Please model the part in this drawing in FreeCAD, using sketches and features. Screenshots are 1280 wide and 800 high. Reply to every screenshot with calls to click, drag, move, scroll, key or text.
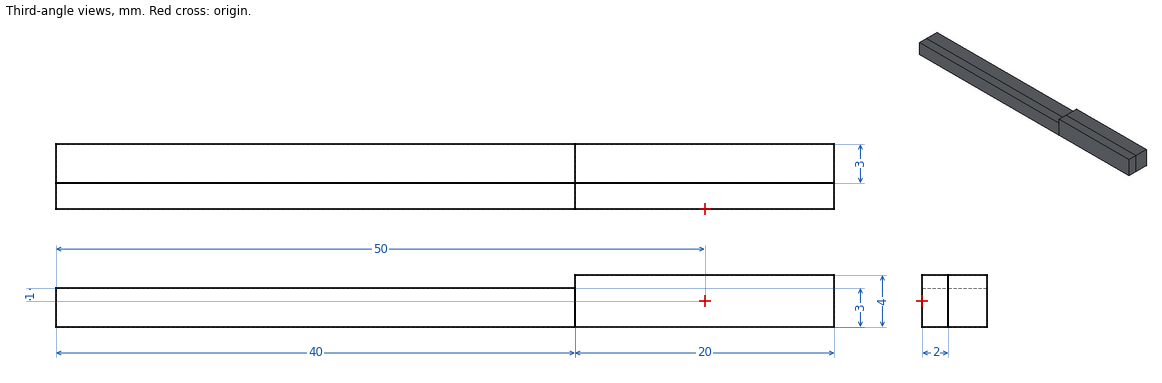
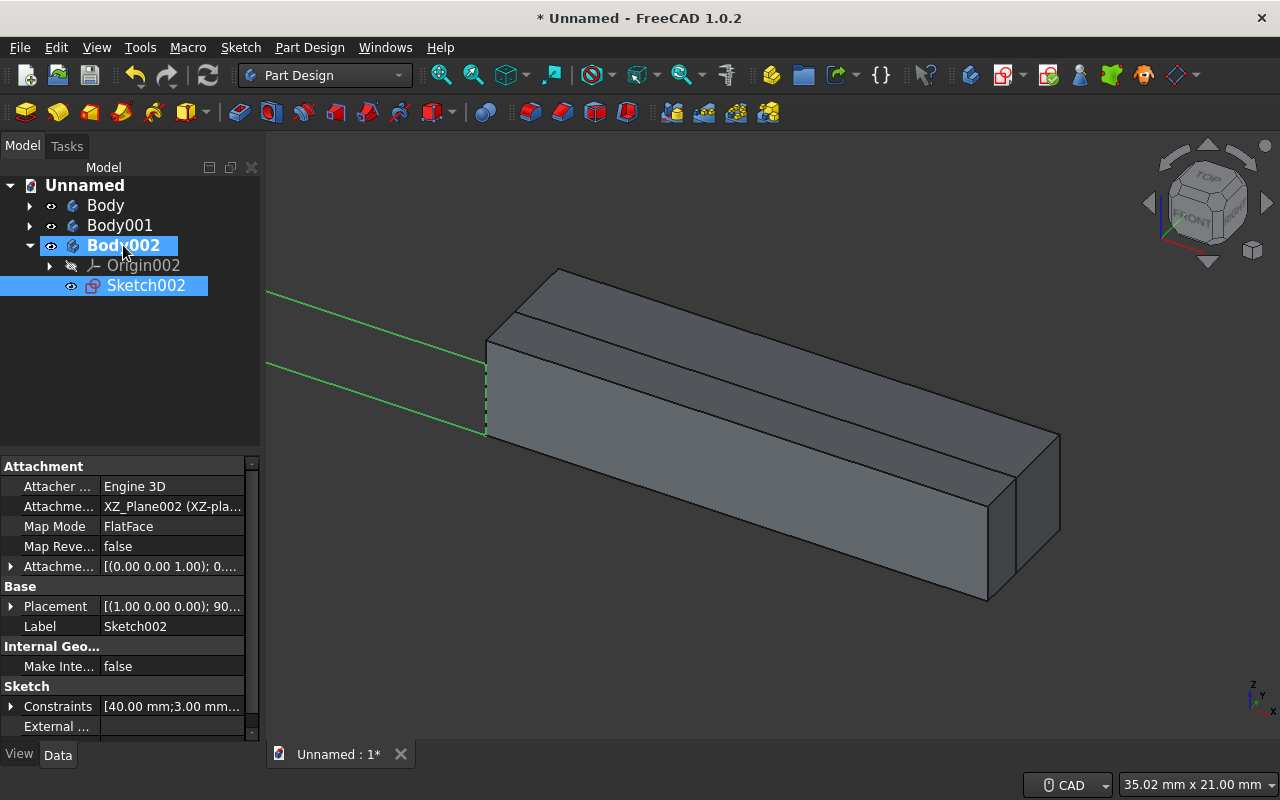
click(26, 112)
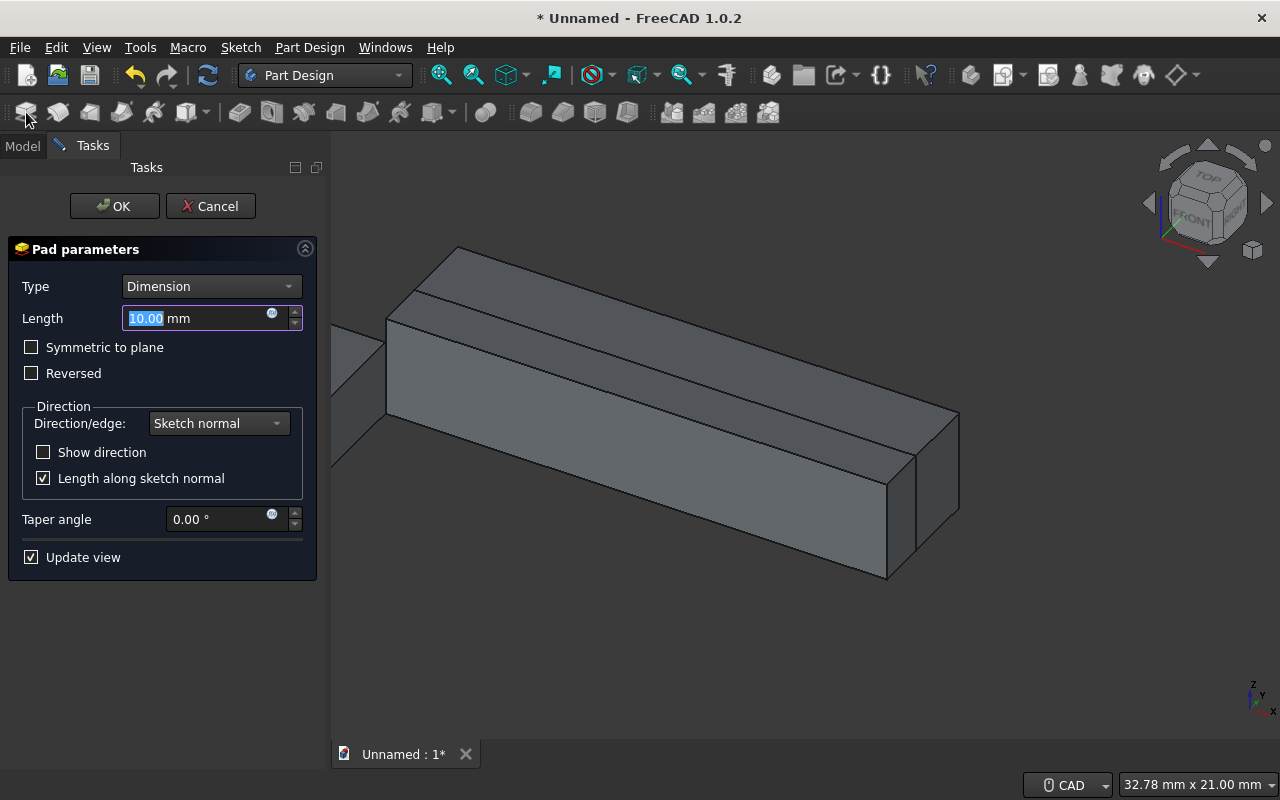
text(2)
key(Tab)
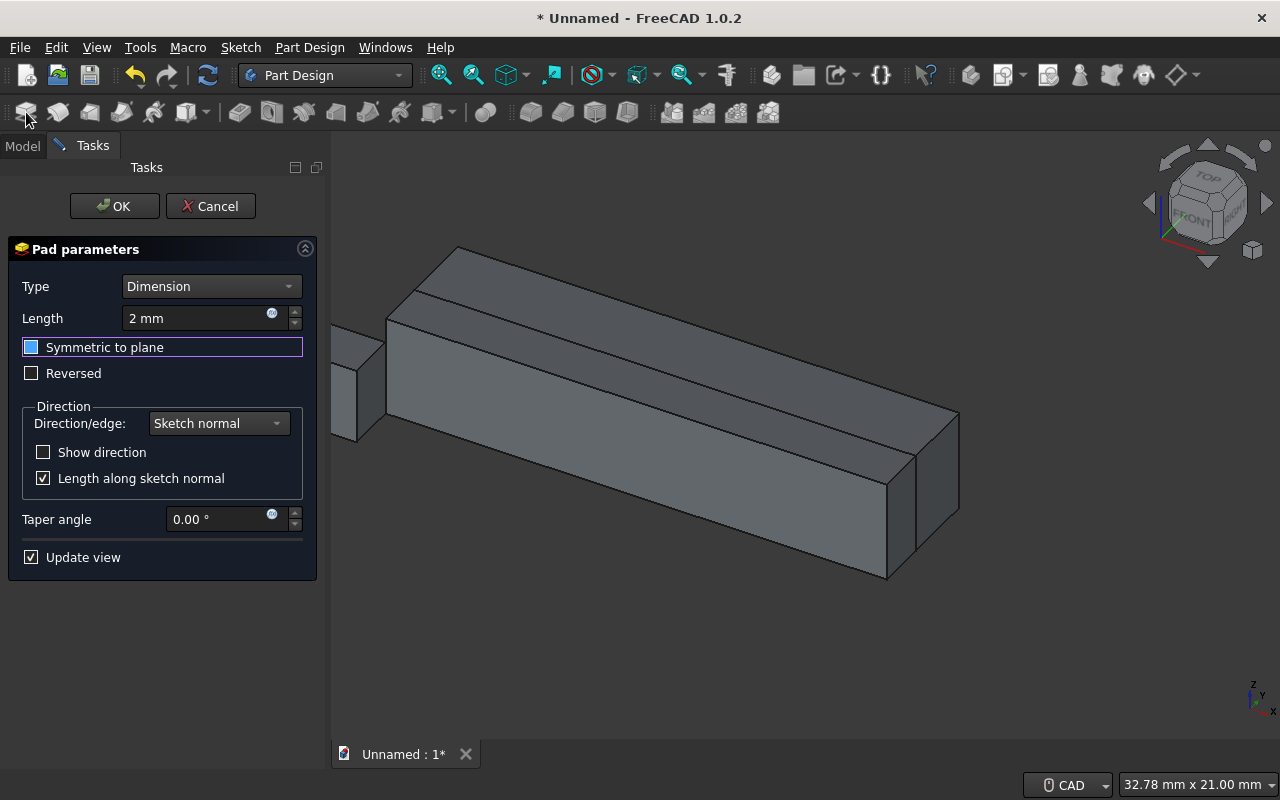
click(30, 373)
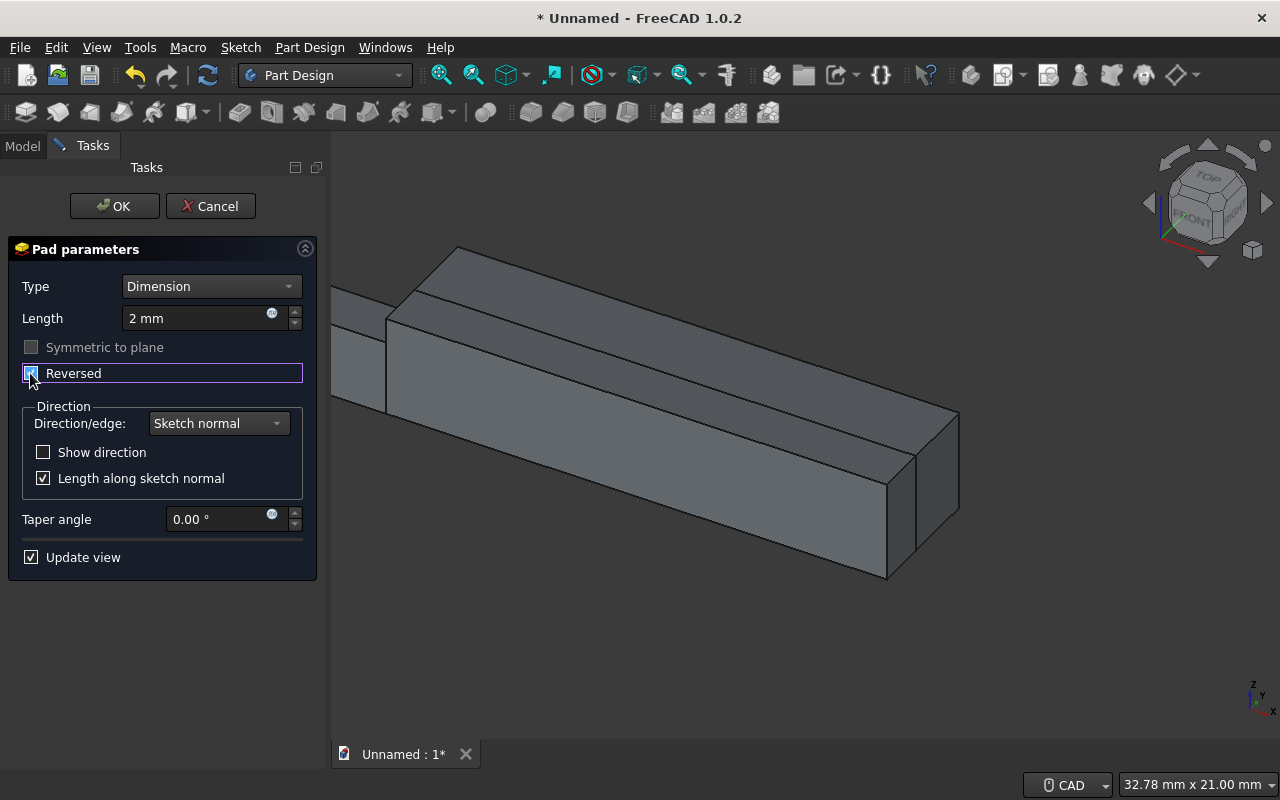
click(115, 206)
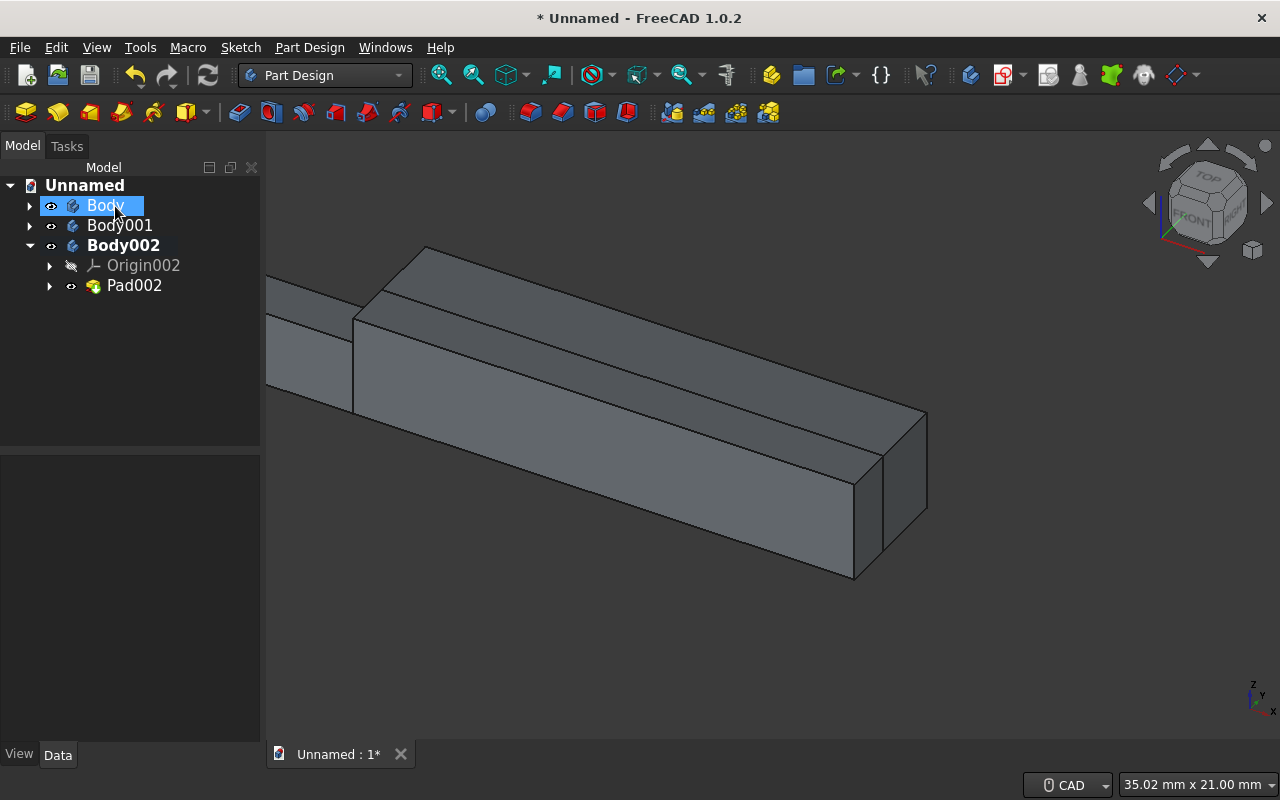
click(442, 76)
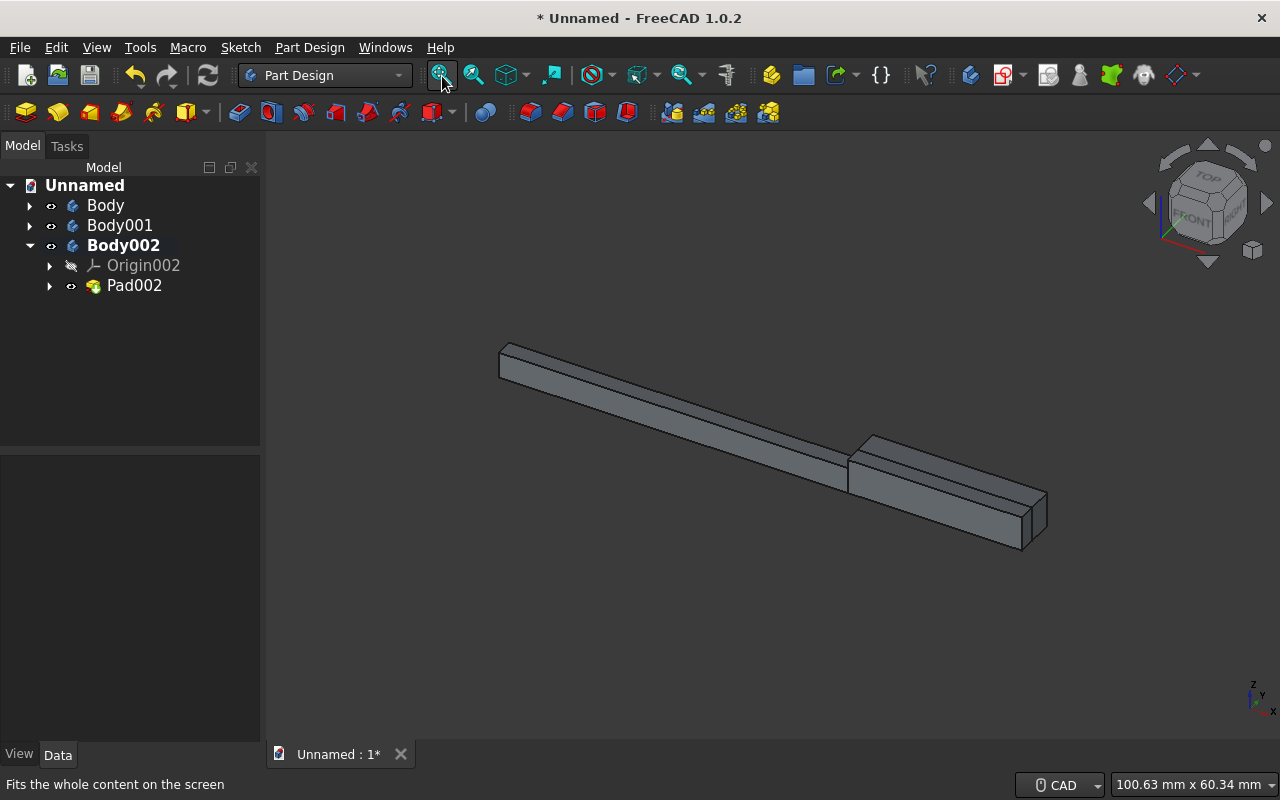
click(972, 76)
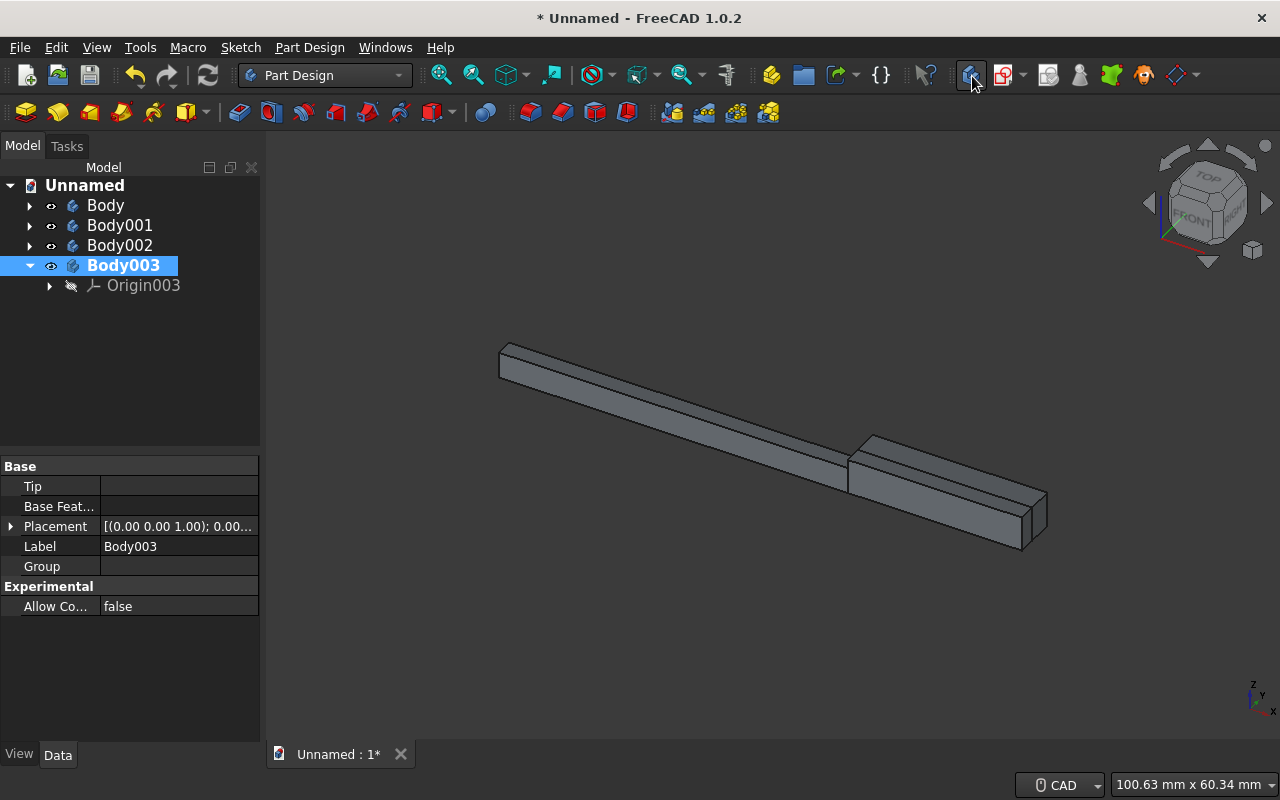
click(50, 286)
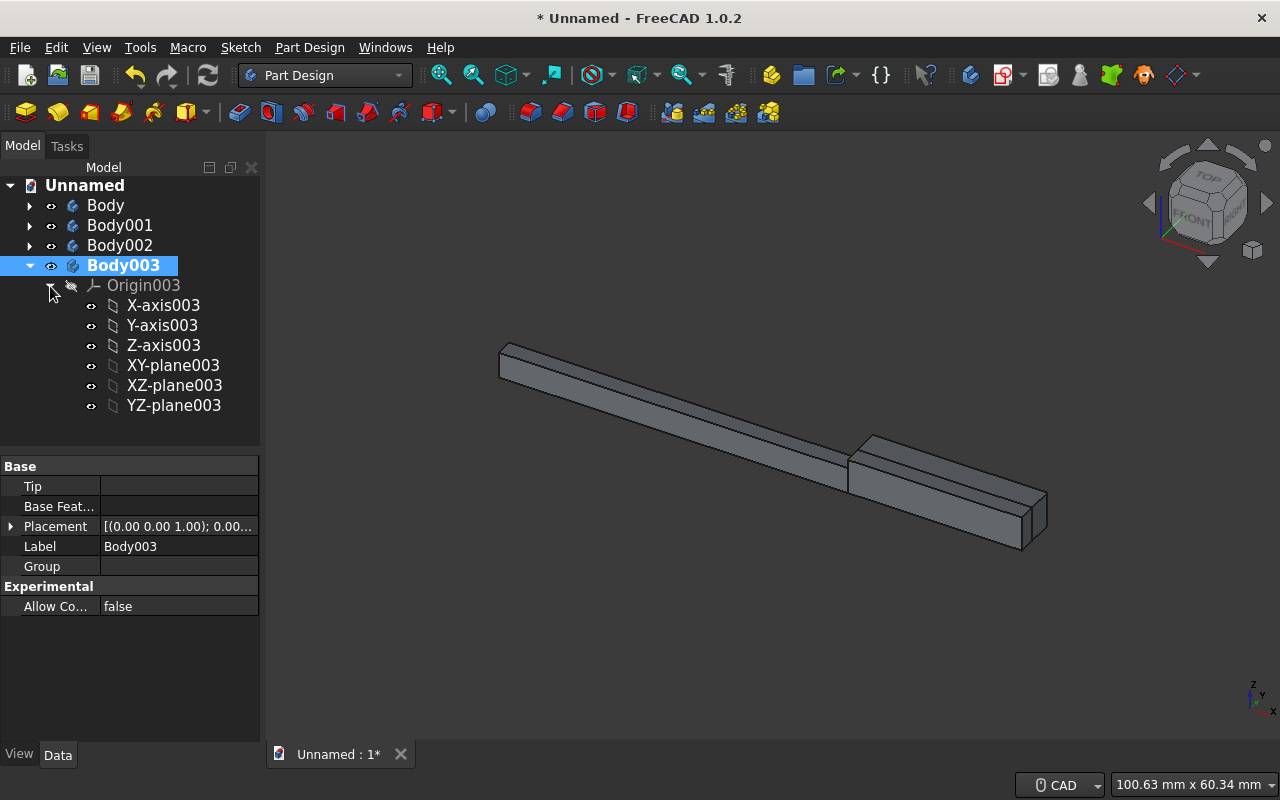
click(136, 386)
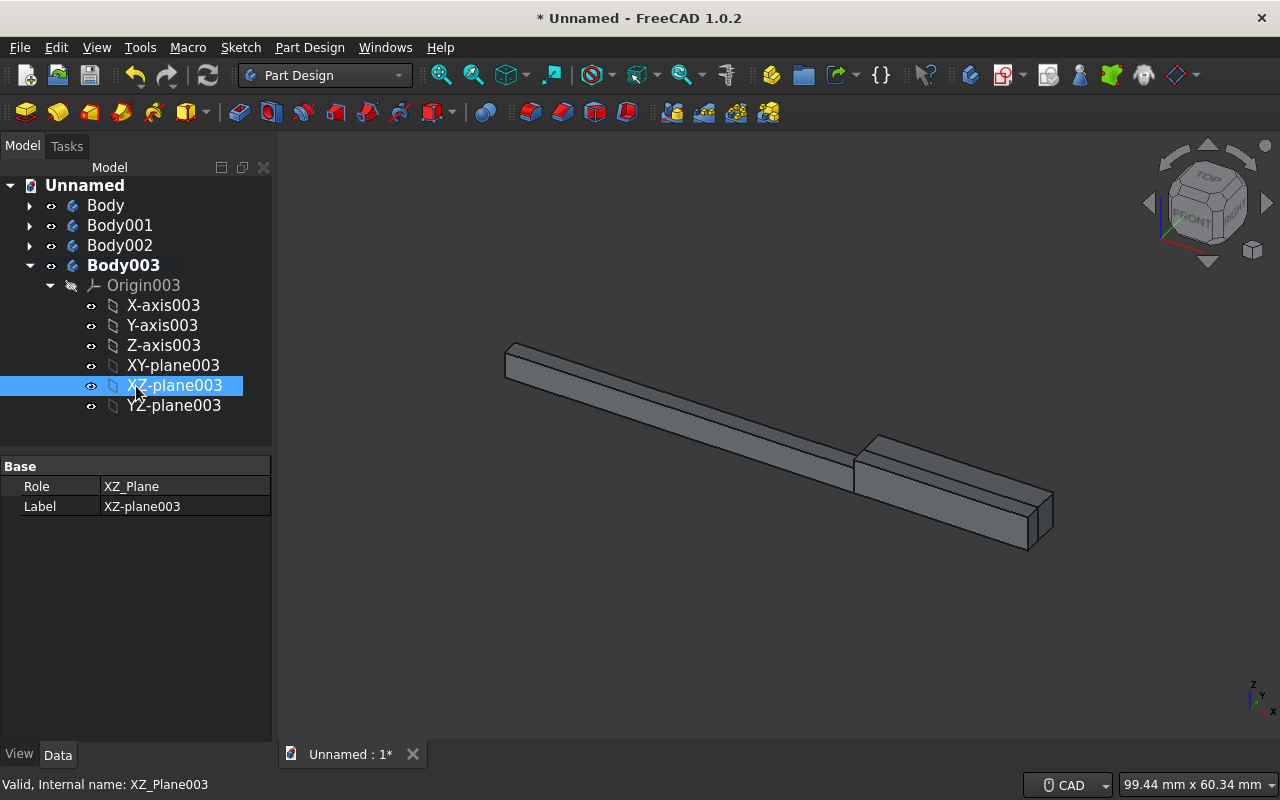
click(1176, 76)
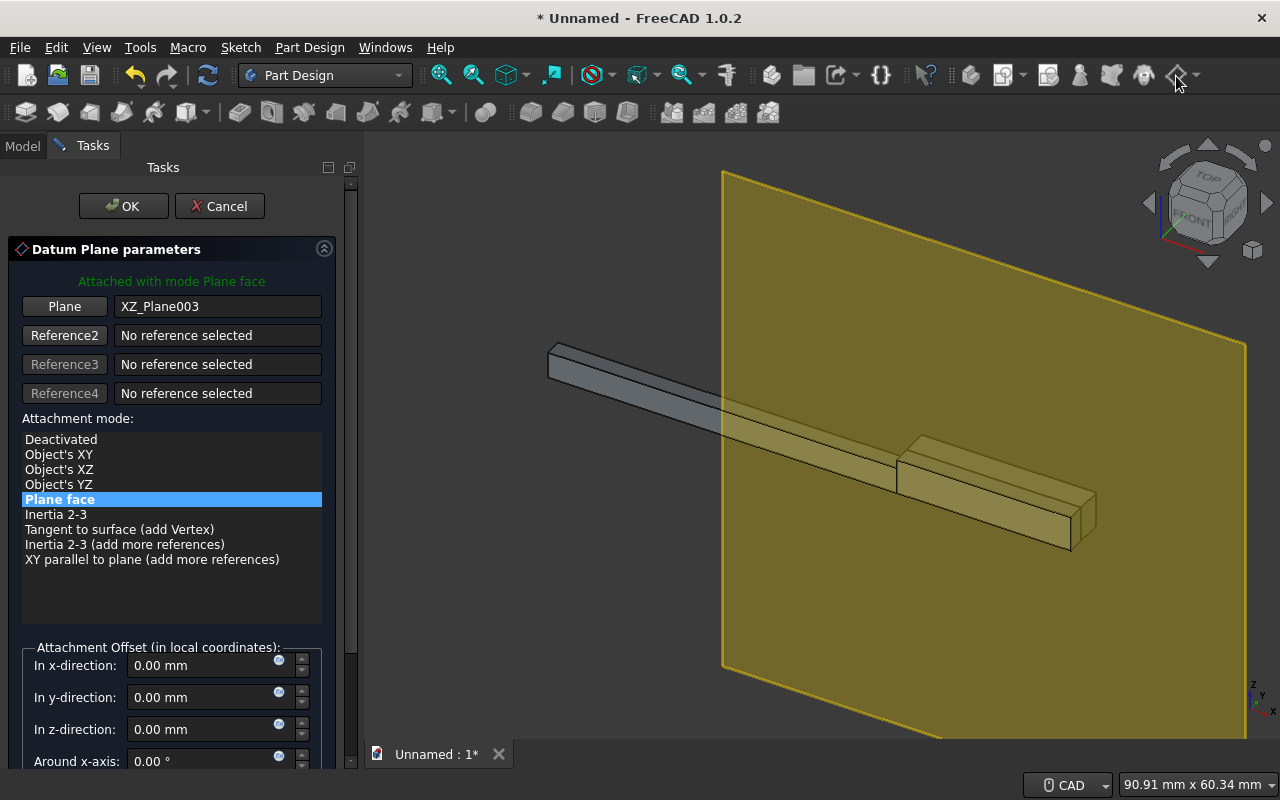
triple_click(210, 729)